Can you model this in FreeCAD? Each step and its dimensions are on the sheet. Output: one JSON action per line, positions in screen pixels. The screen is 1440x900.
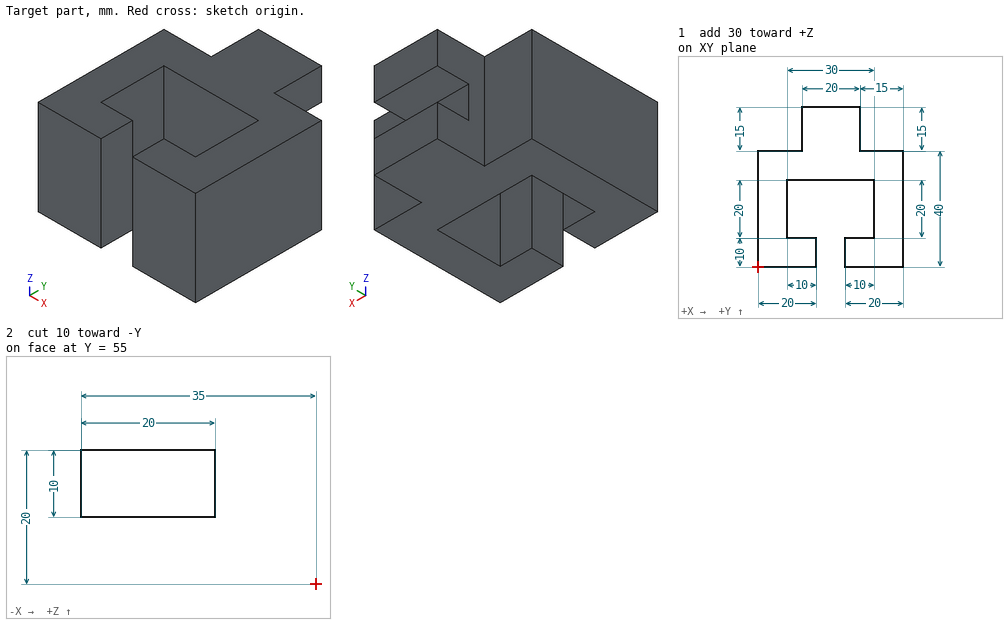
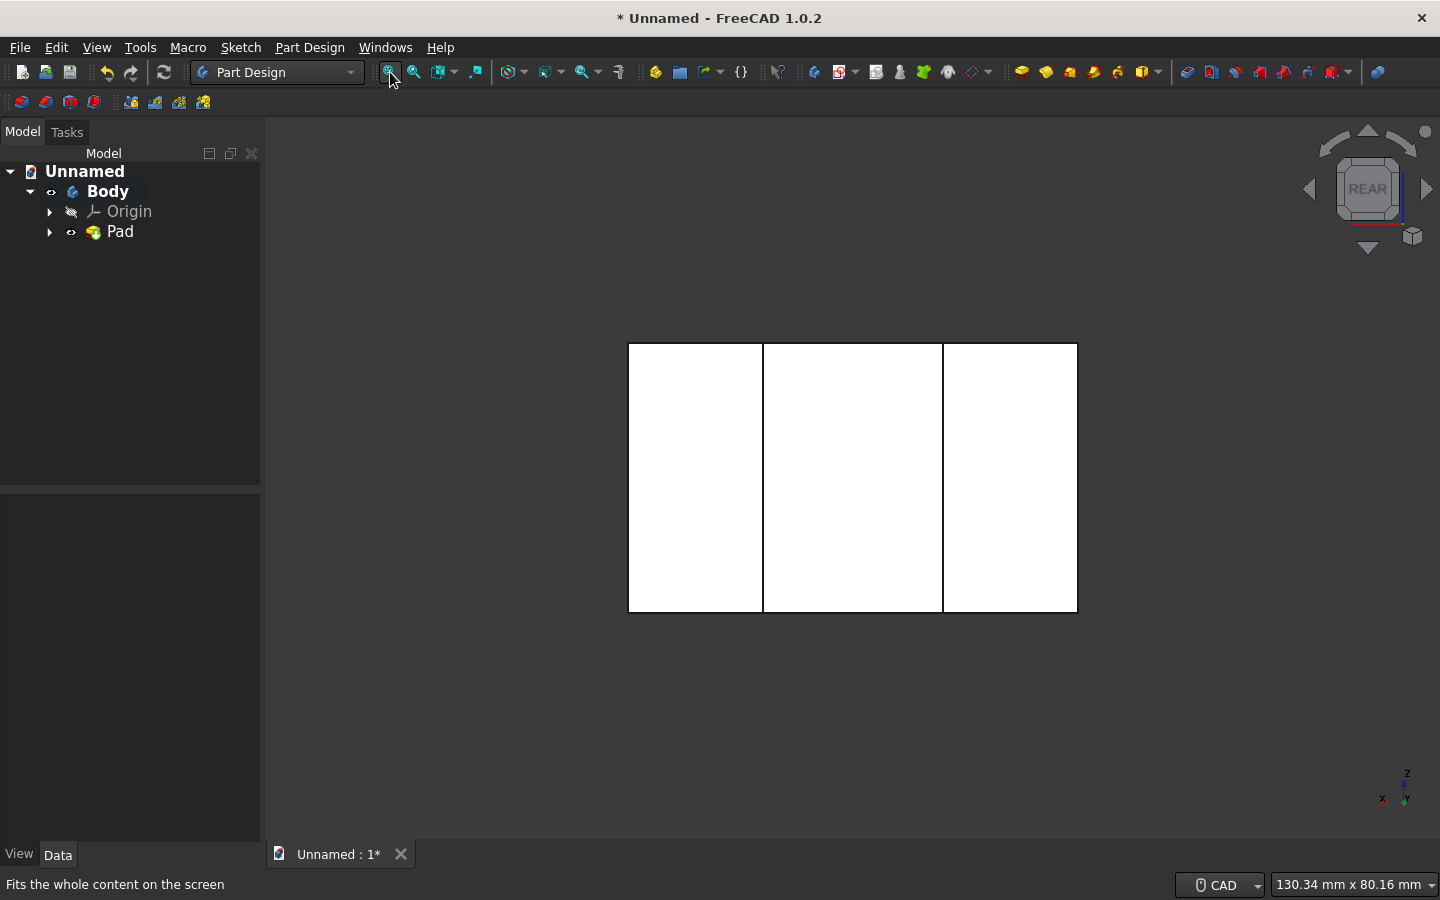
{"action": "left_click", "coordinate": [853, 438]}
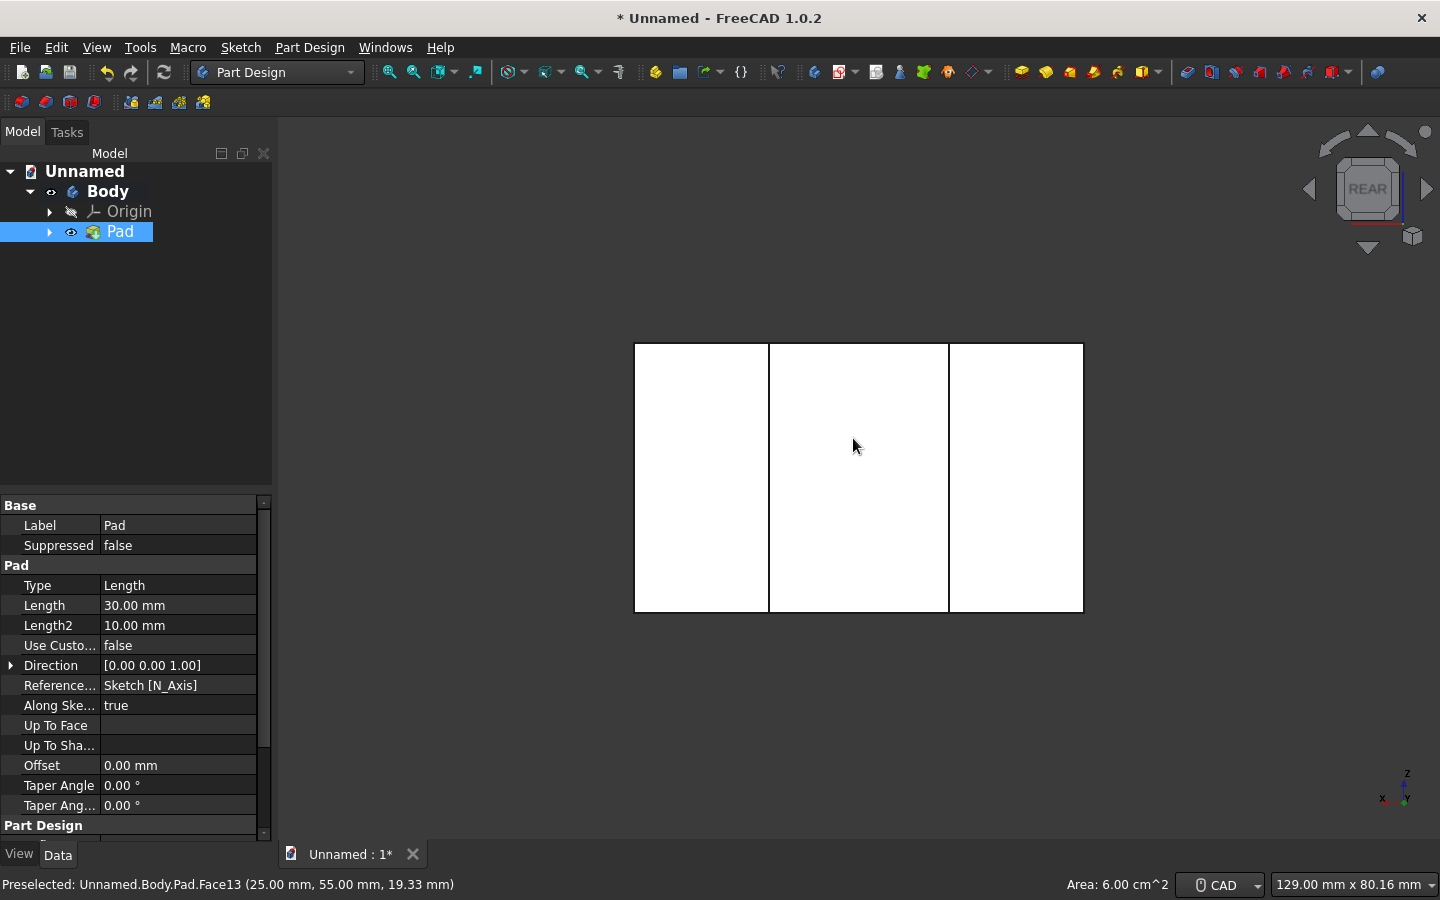
{"action": "left_click", "coordinate": [840, 72]}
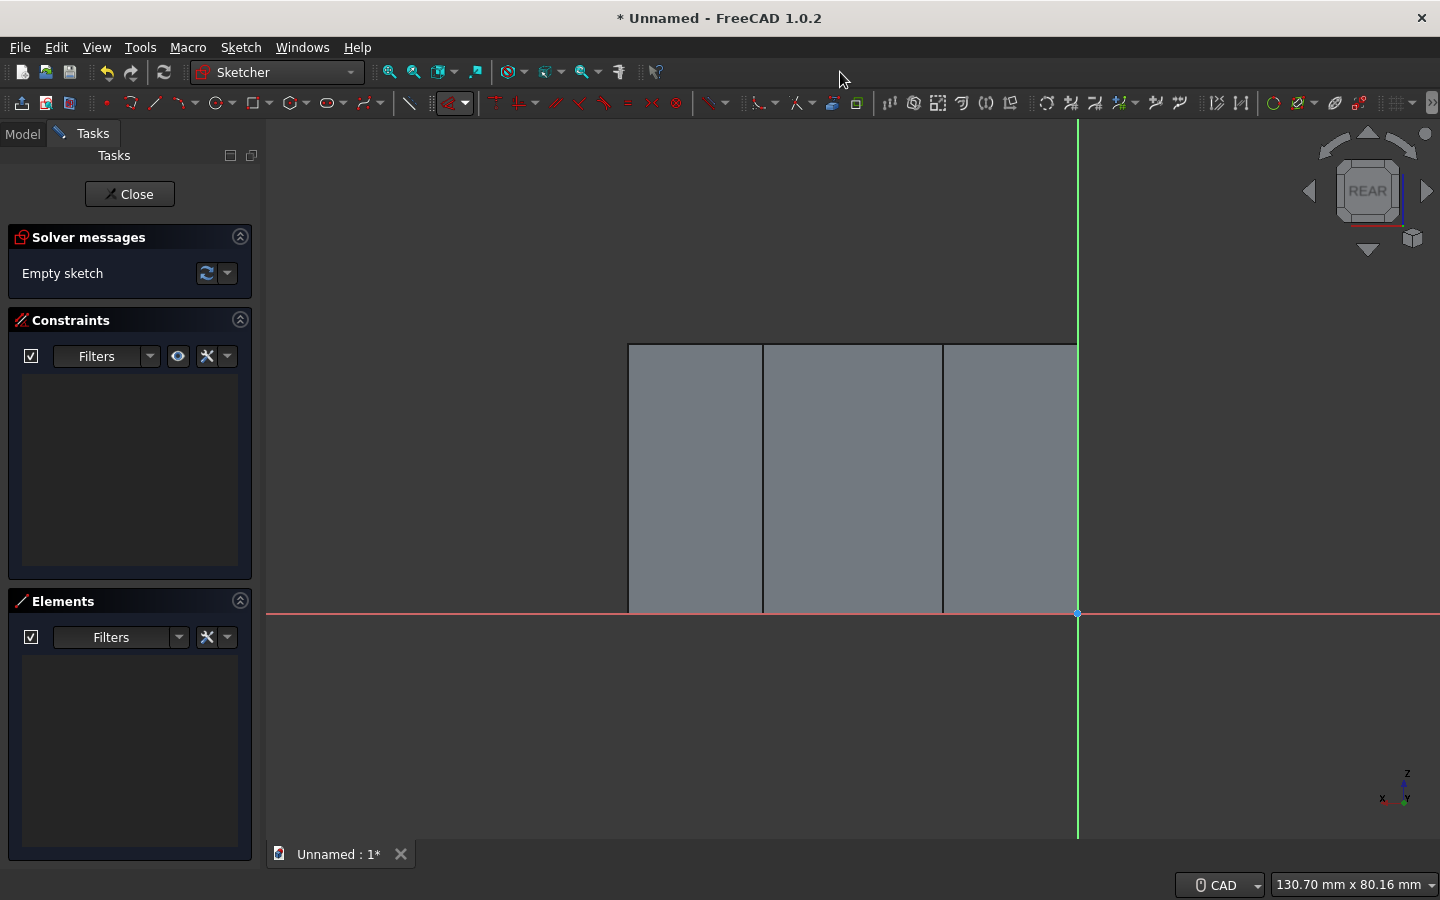
{"action": "scroll", "coordinate": [1031, 561], "scroll_direction": "up", "scroll_amount": 4}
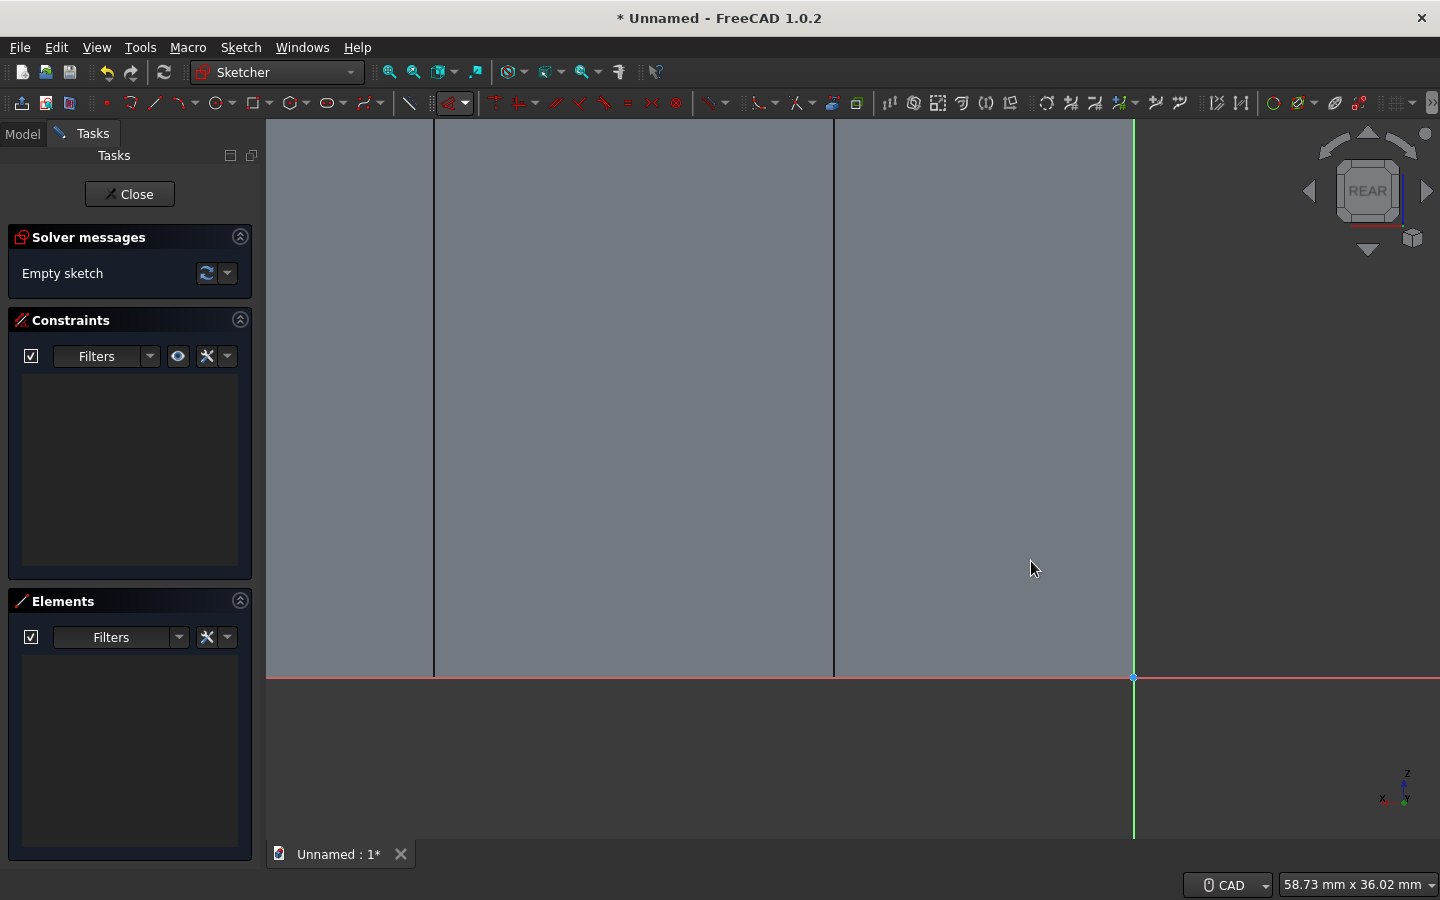
{"action": "key", "text": "g r"}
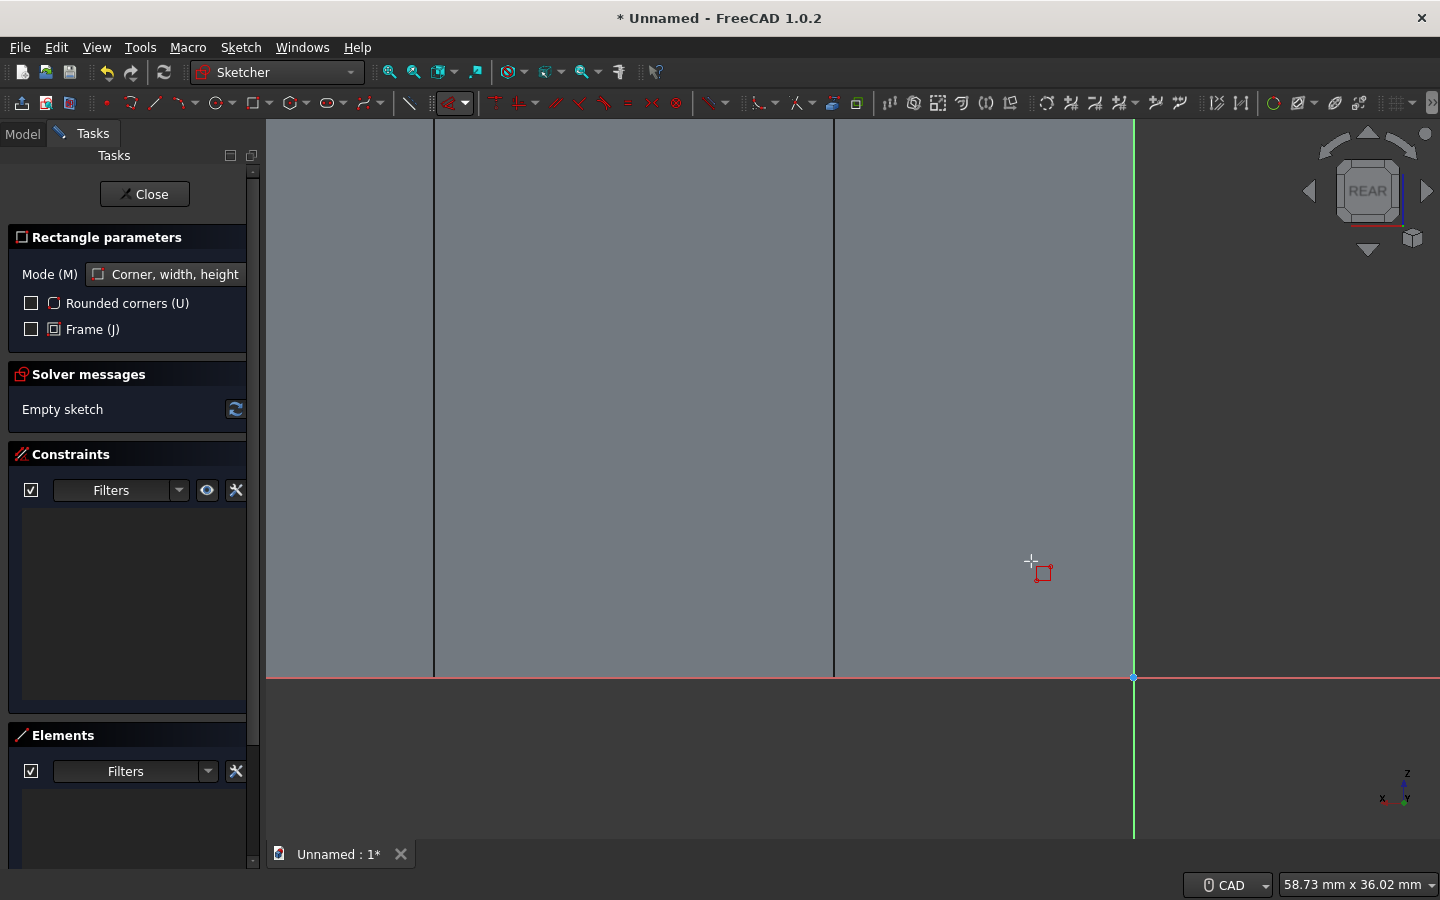
{"action": "left_click", "coordinate": [434, 278]}
{"action": "left_click", "coordinate": [834, 478]}
{"action": "key", "text": "Escape"}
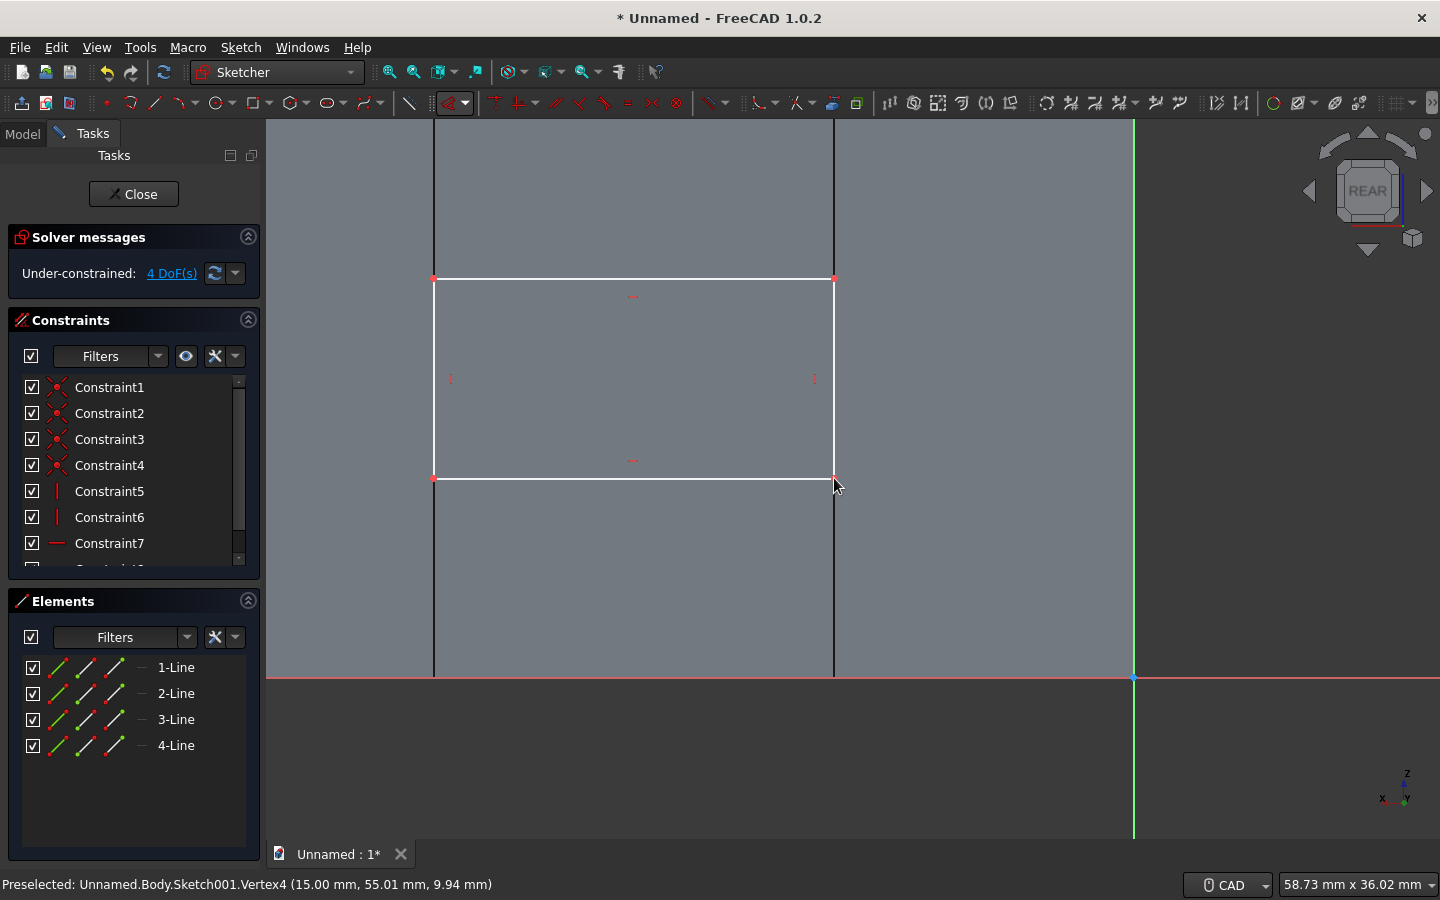
{"action": "left_click", "coordinate": [448, 104]}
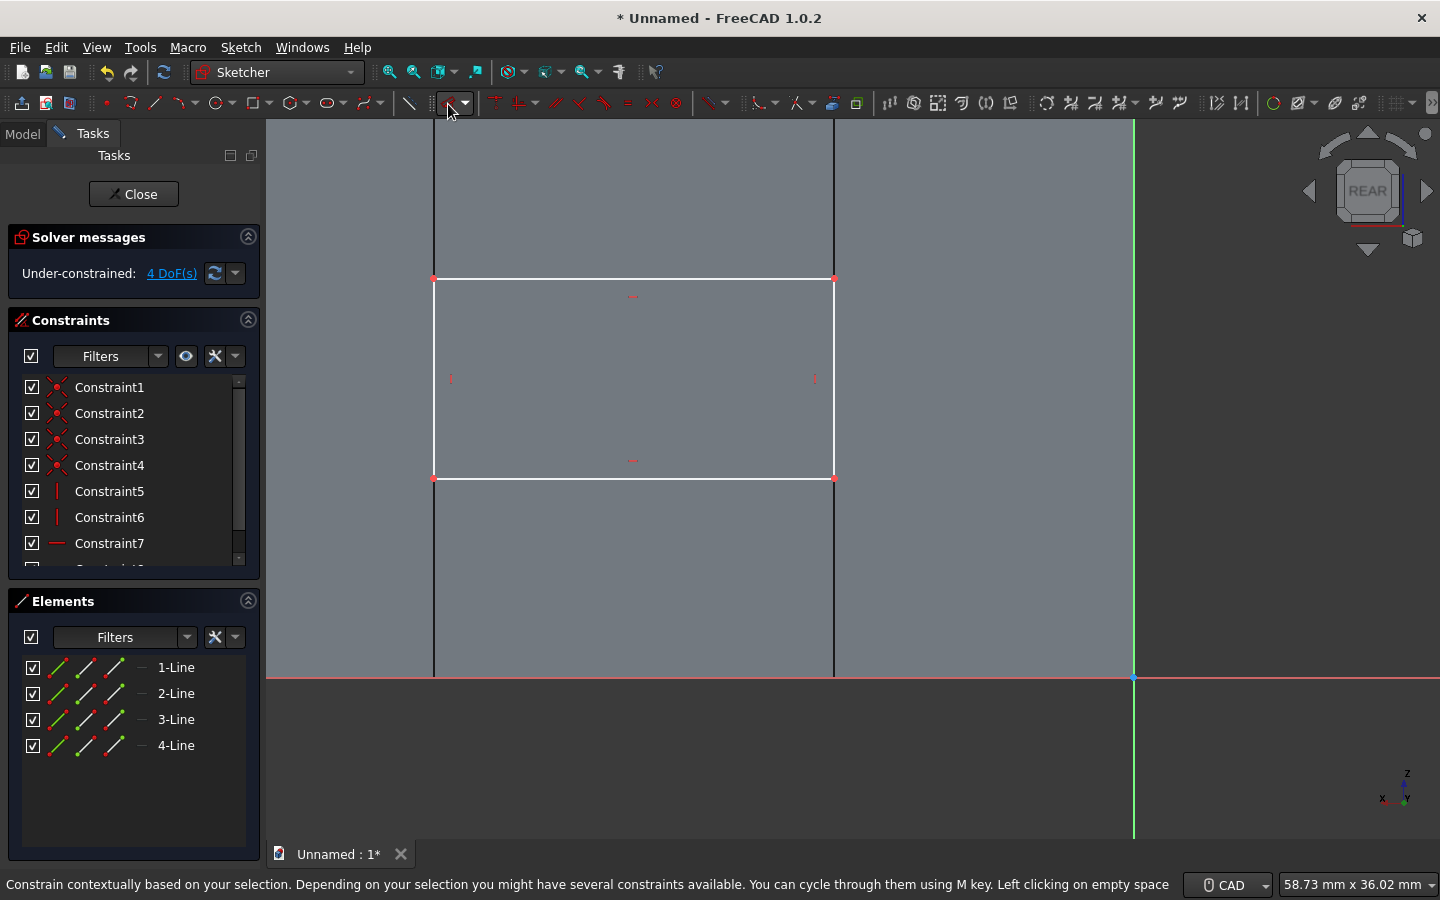
{"action": "left_click", "coordinate": [434, 339]}
{"action": "left_click", "coordinate": [400, 379]}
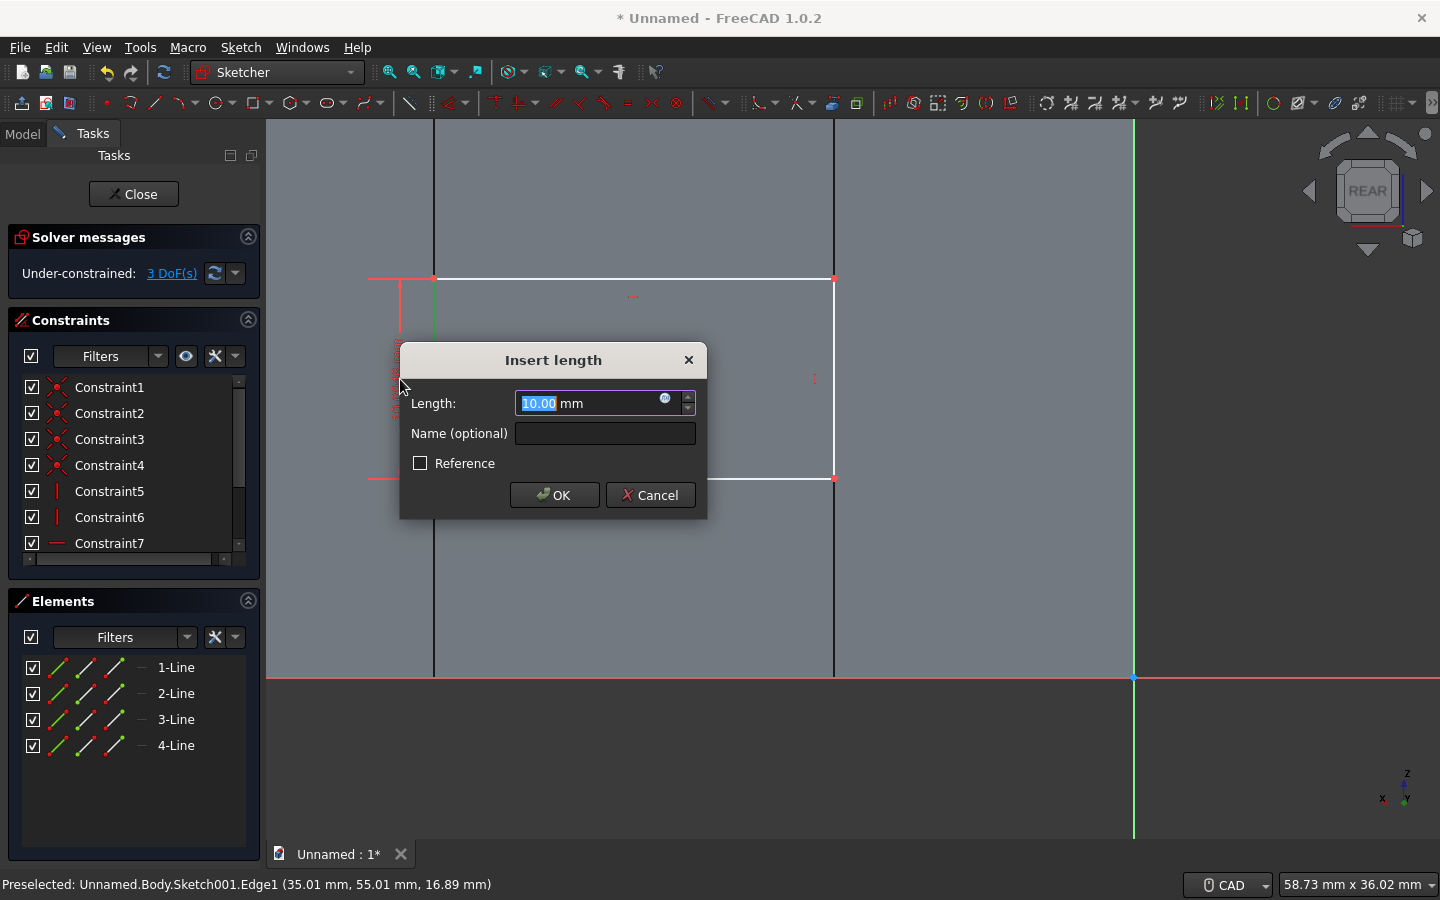
{"action": "type", "text": "10"}
{"action": "key", "text": "Return"}